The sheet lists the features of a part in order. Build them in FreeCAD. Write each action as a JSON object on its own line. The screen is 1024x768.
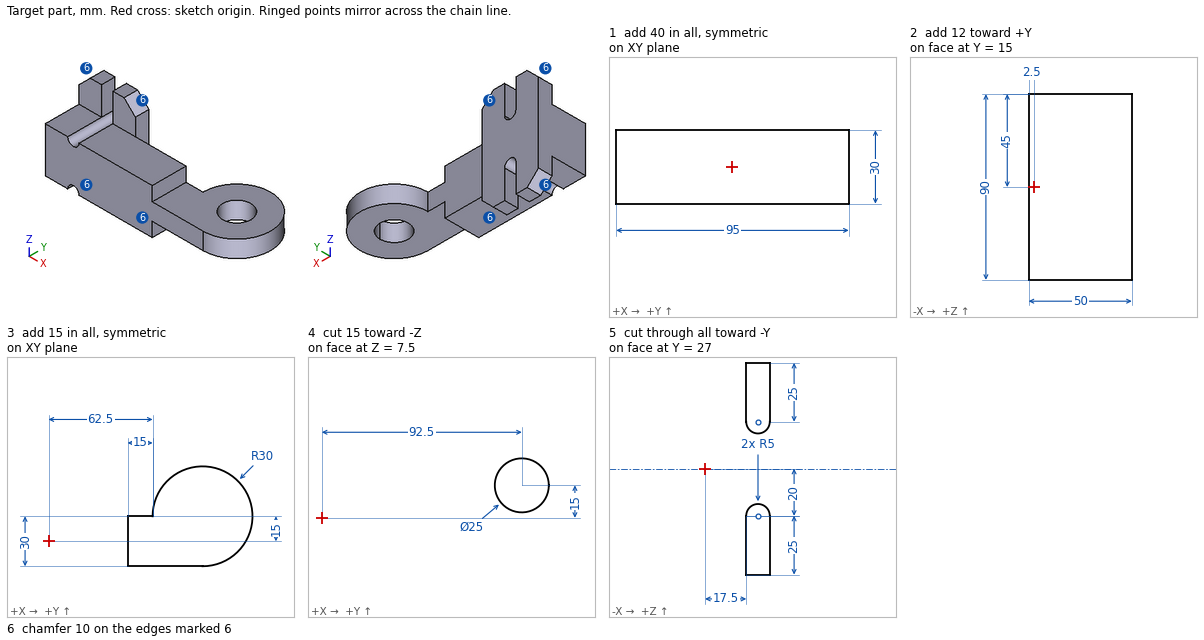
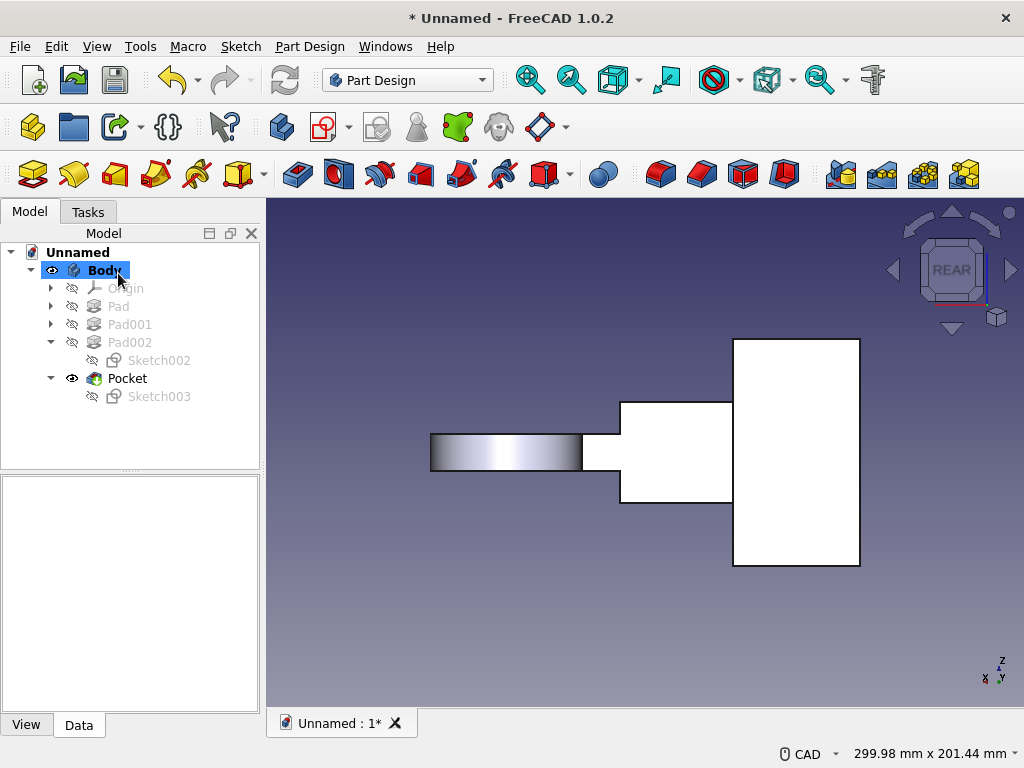
{"action": "left_click", "coordinate": [797, 419]}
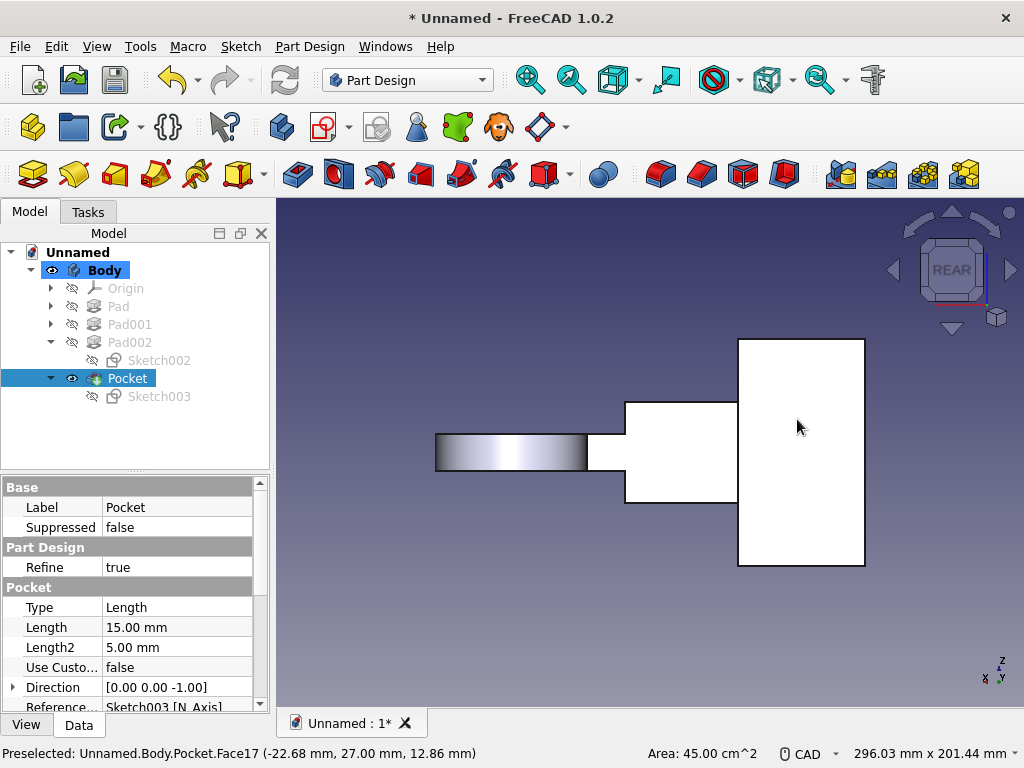
{"action": "left_click", "coordinate": [322, 128]}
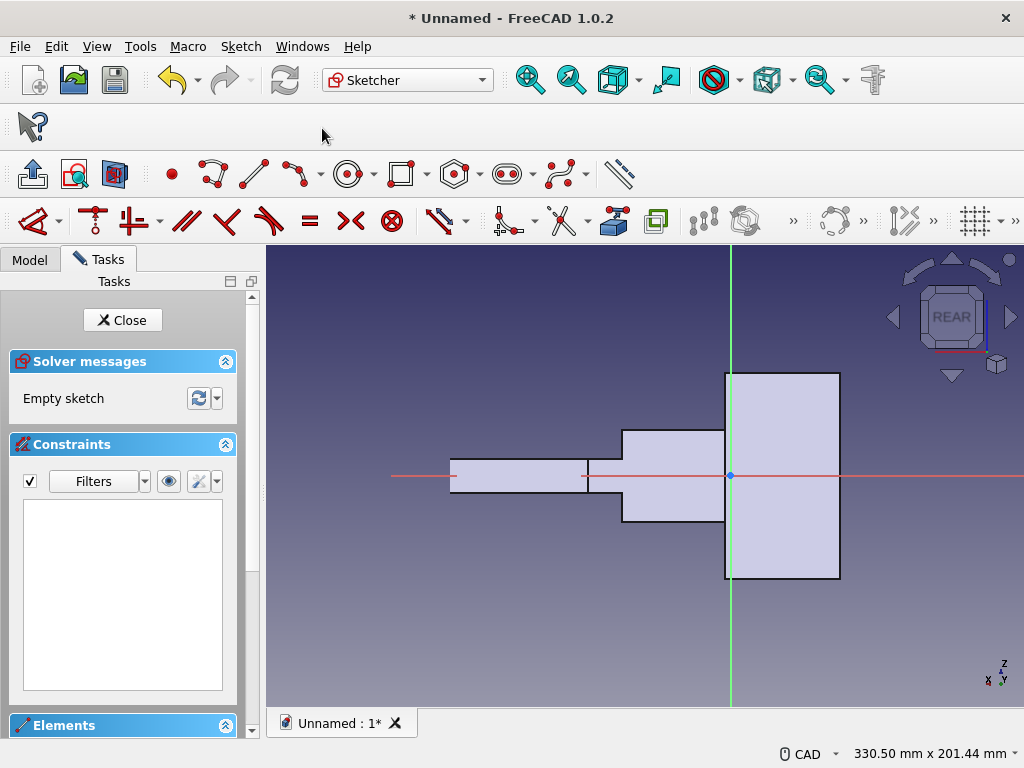
{"action": "left_click", "coordinate": [115, 174]}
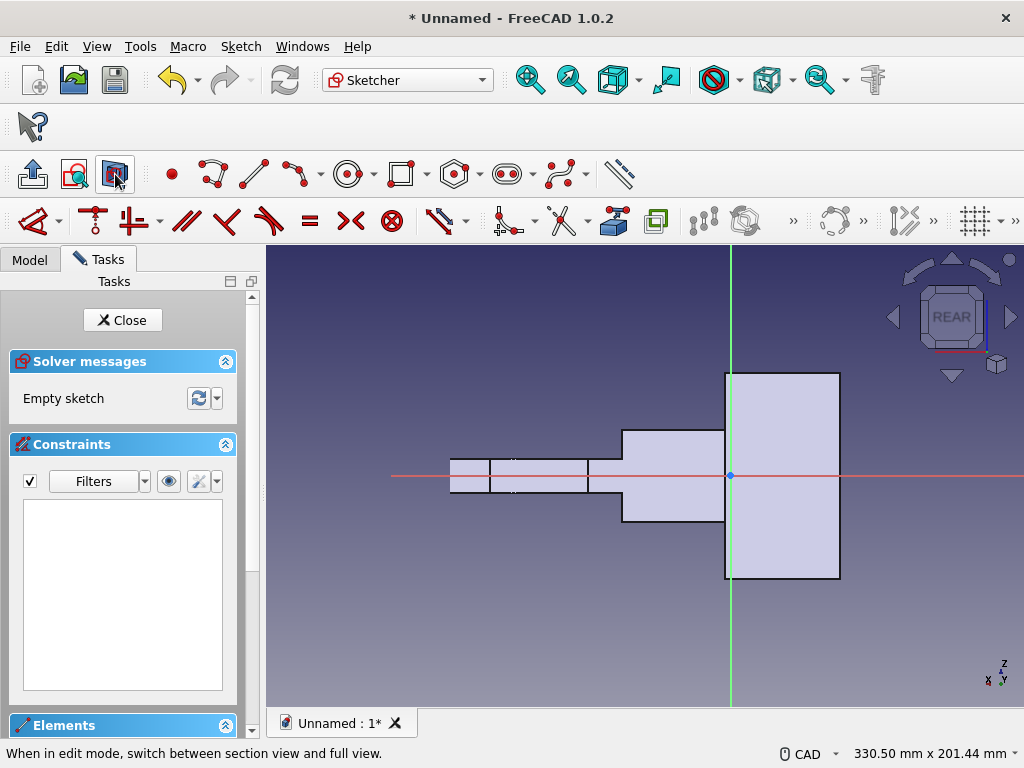
{"action": "scroll", "coordinate": [859, 476], "scroll_direction": "up", "scroll_amount": 2}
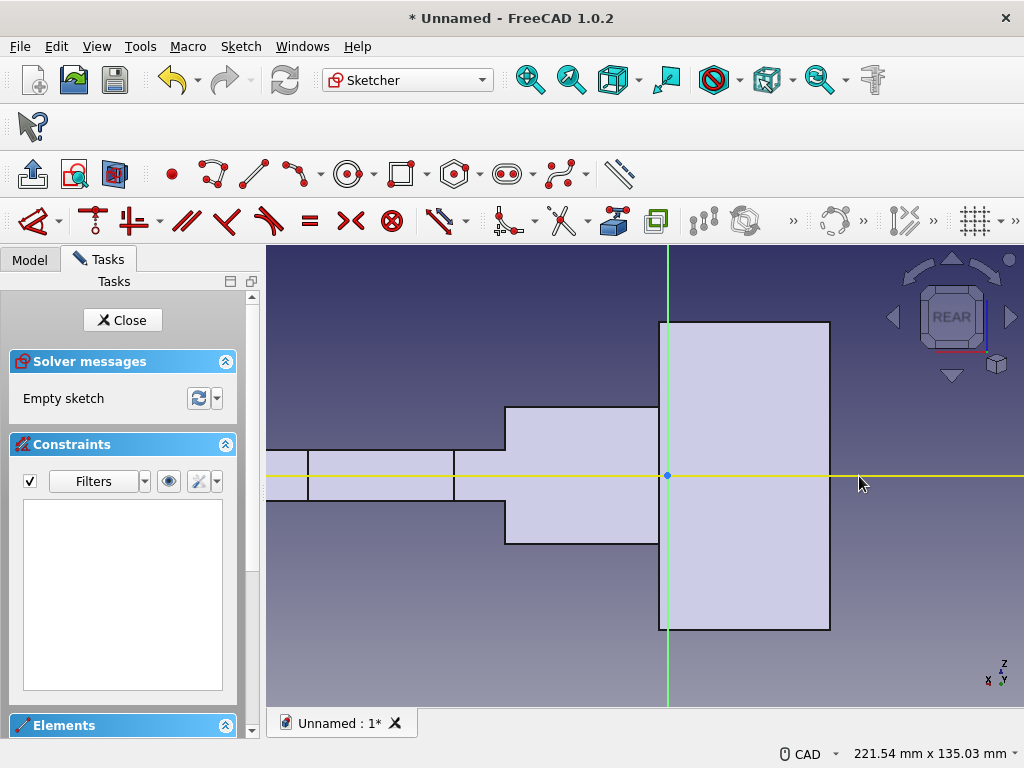
{"action": "left_click", "coordinate": [213, 174]}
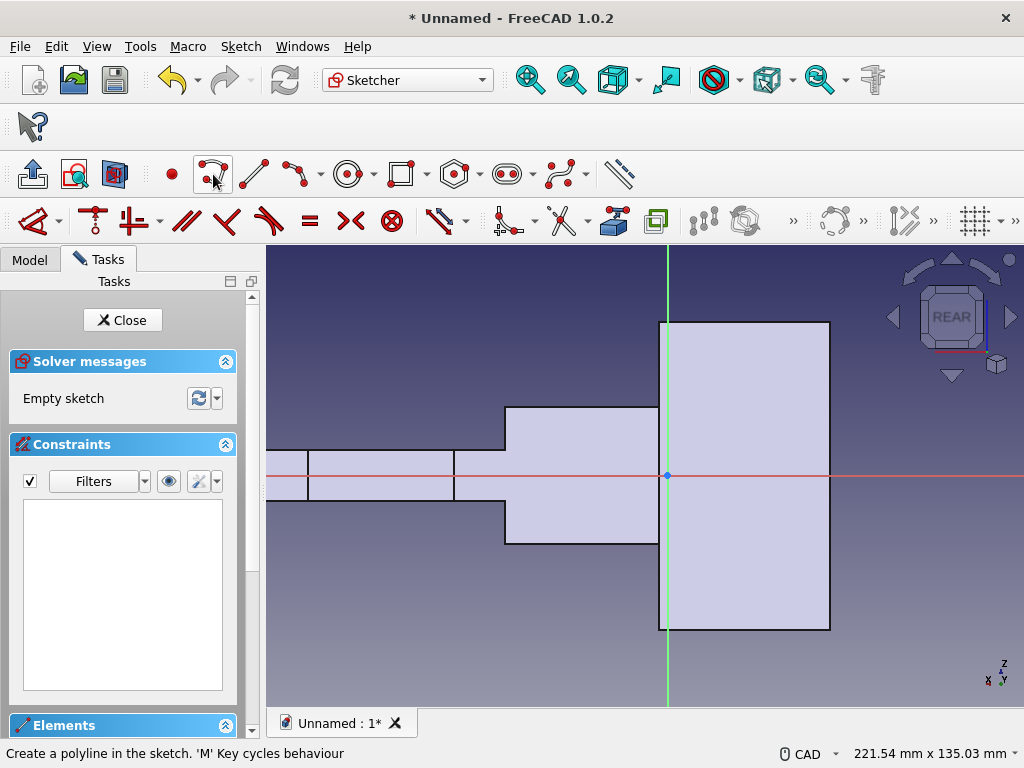
{"action": "left_click", "coordinate": [727, 544]}
{"action": "left_click", "coordinate": [727, 630]}
{"action": "left_click", "coordinate": [762, 630]}
{"action": "left_click", "coordinate": [762, 544]}
{"action": "right_click", "coordinate": [762, 544]}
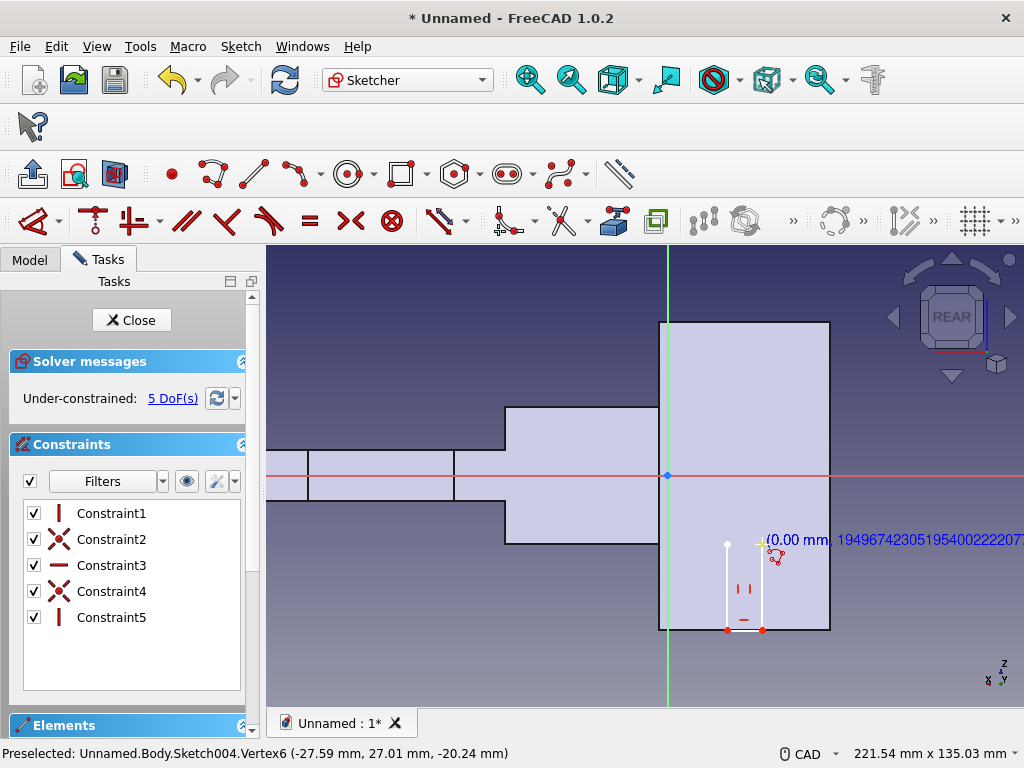
{"action": "left_click", "coordinate": [294, 174]}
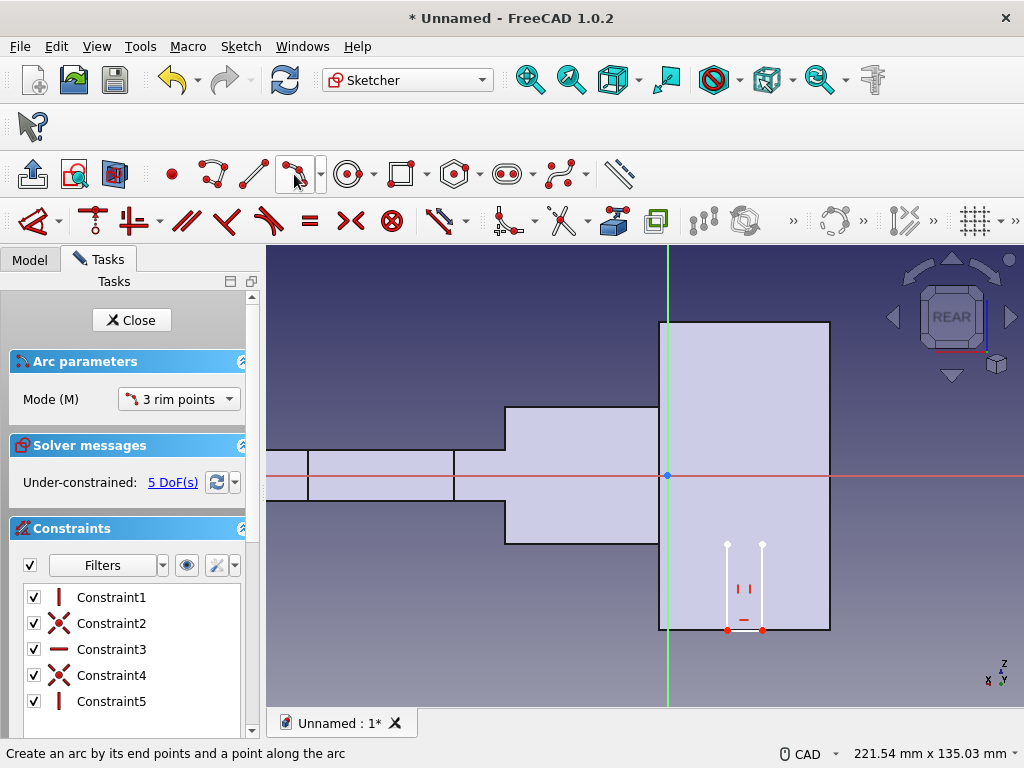
{"action": "left_click", "coordinate": [762, 545]}
{"action": "left_click", "coordinate": [727, 545]}
{"action": "left_click", "coordinate": [745, 527]}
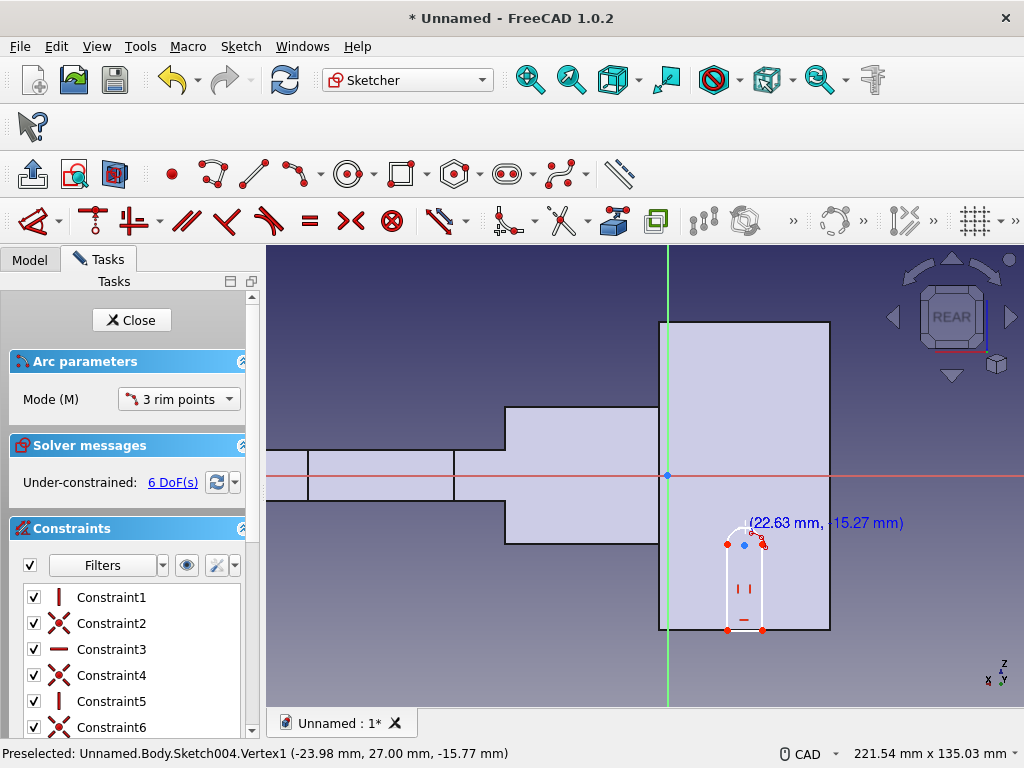
{"action": "left_click", "coordinate": [213, 174]}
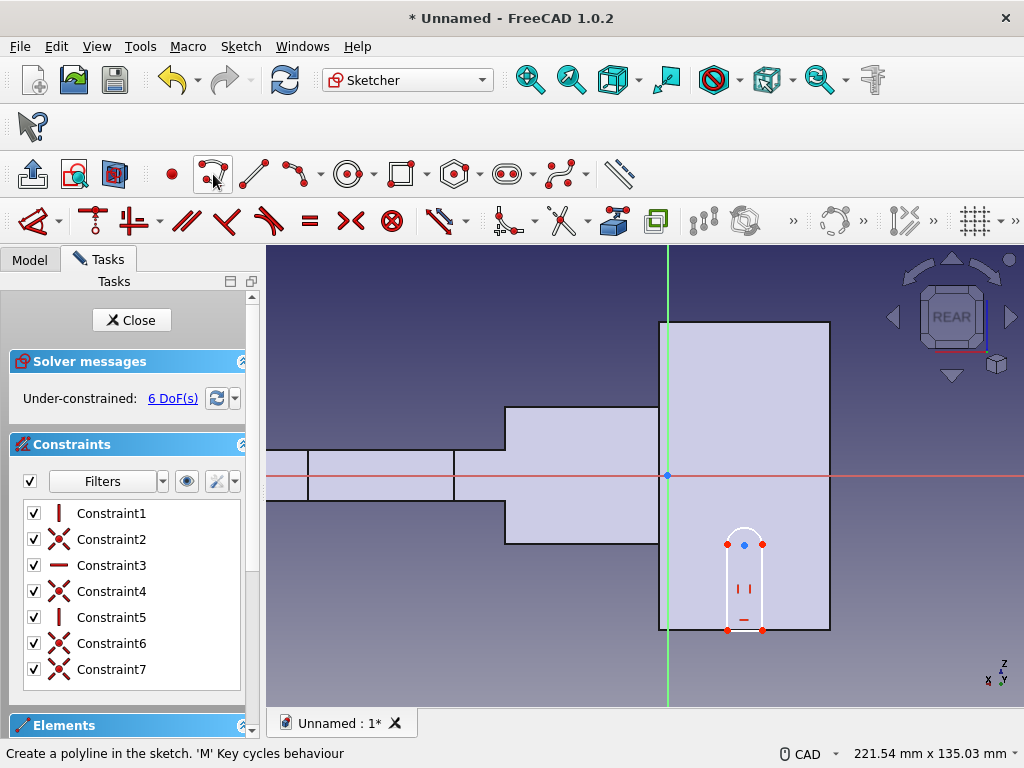
{"action": "left_click", "coordinate": [762, 407]}
{"action": "left_click", "coordinate": [762, 322]}
{"action": "left_click", "coordinate": [727, 322]}
{"action": "left_click", "coordinate": [727, 407]}
{"action": "right_click", "coordinate": [727, 407]}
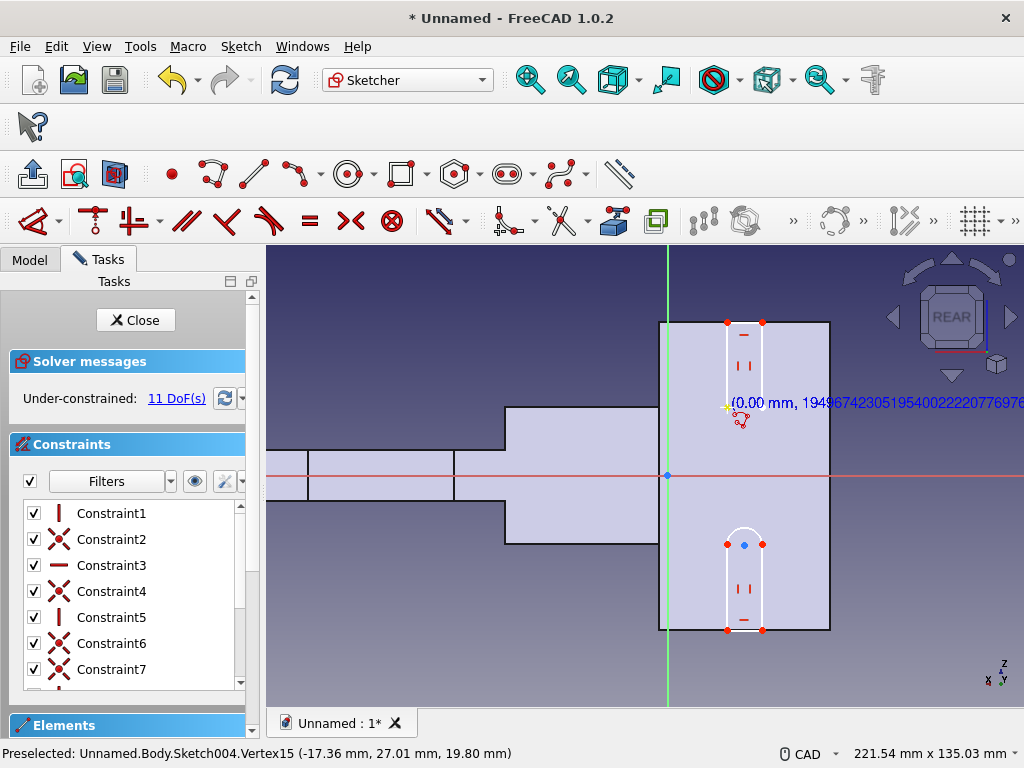
{"action": "key", "text": "g 3 a"}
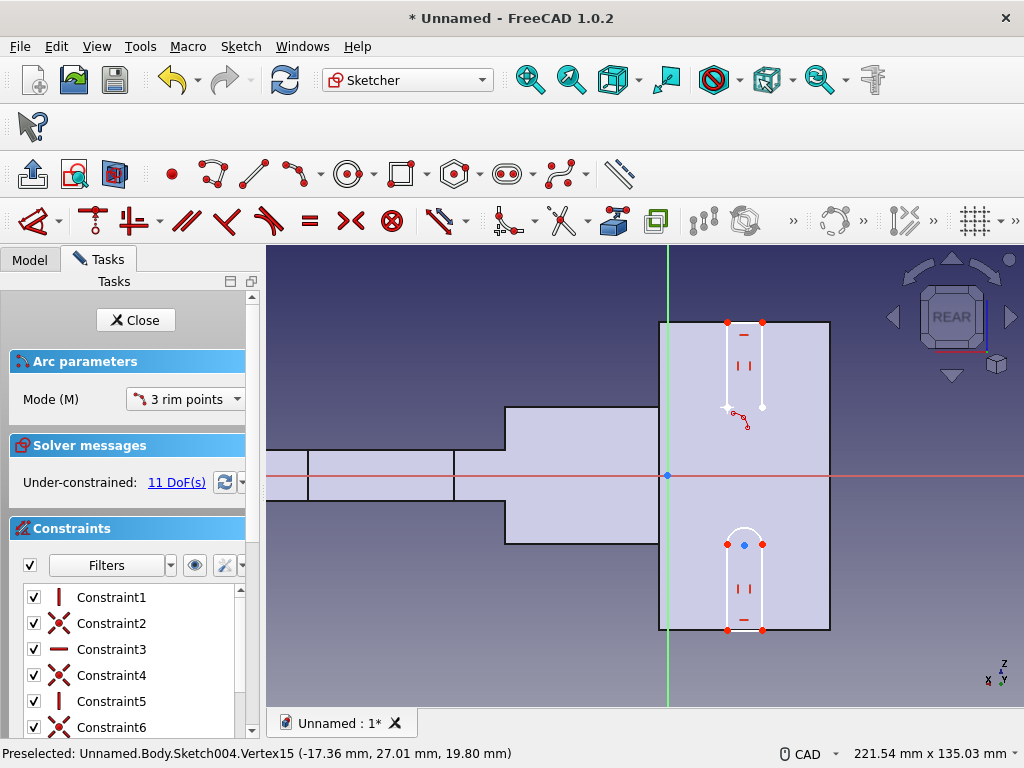
{"action": "left_click", "coordinate": [727, 408]}
{"action": "left_click", "coordinate": [762, 408]}
{"action": "left_click", "coordinate": [745, 424]}
{"action": "key", "text": "Escape"}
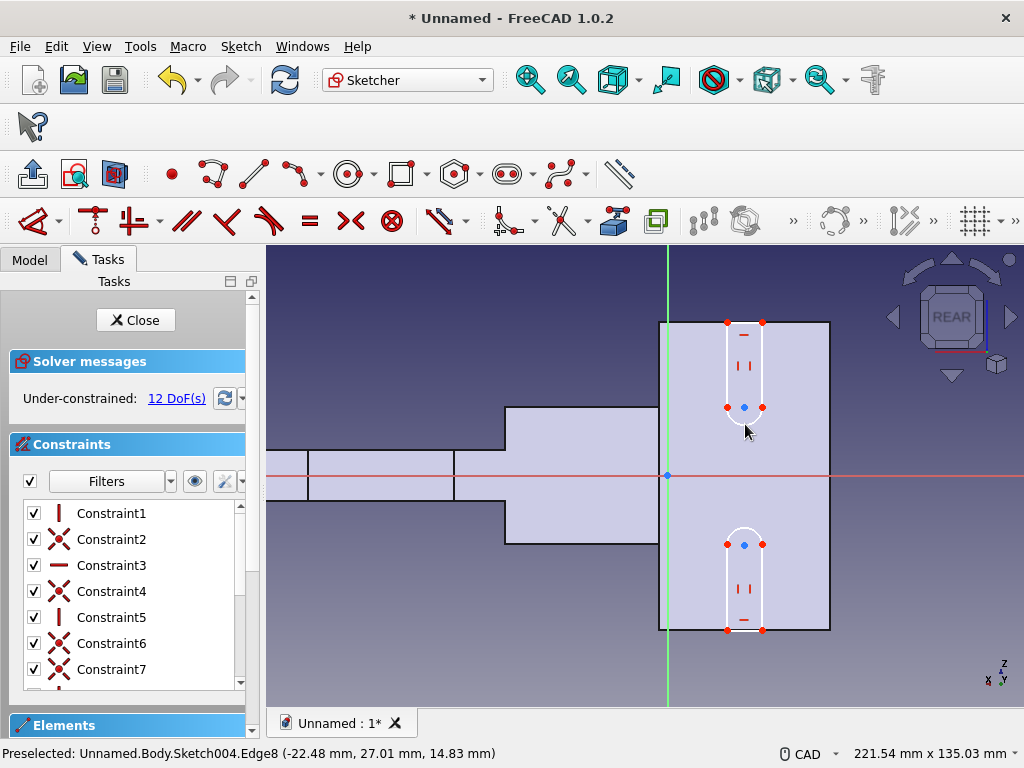
{"action": "left_click", "coordinate": [727, 571]}